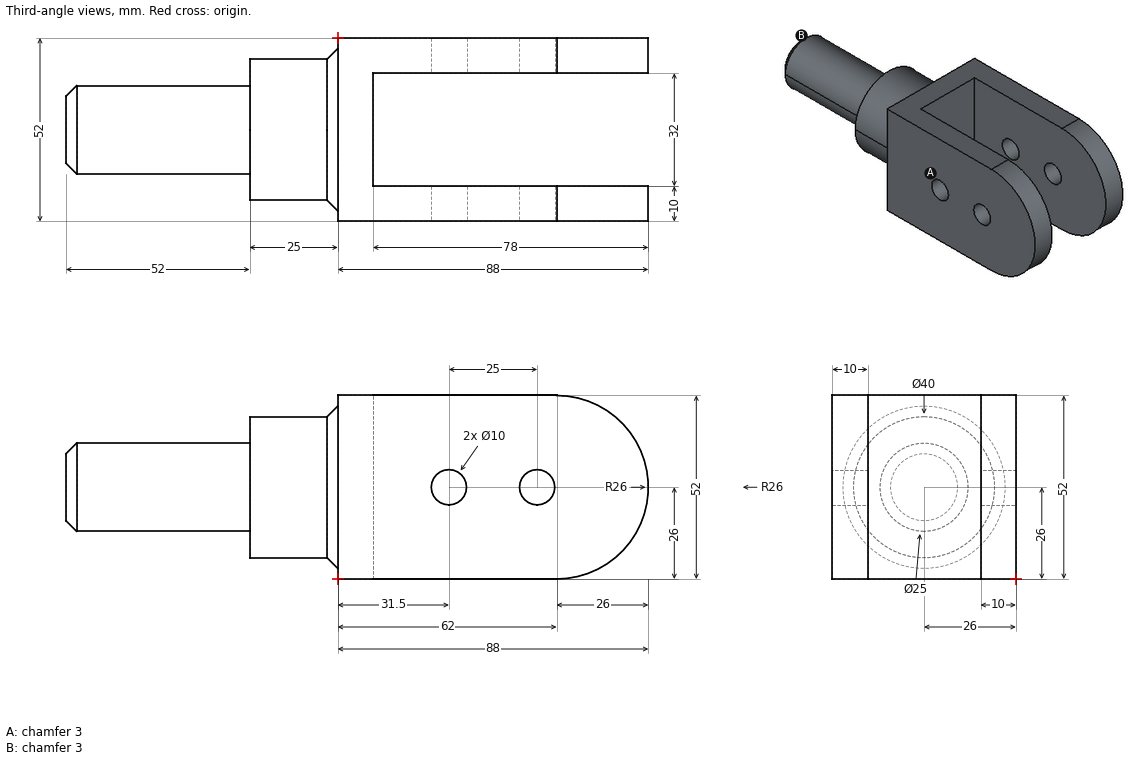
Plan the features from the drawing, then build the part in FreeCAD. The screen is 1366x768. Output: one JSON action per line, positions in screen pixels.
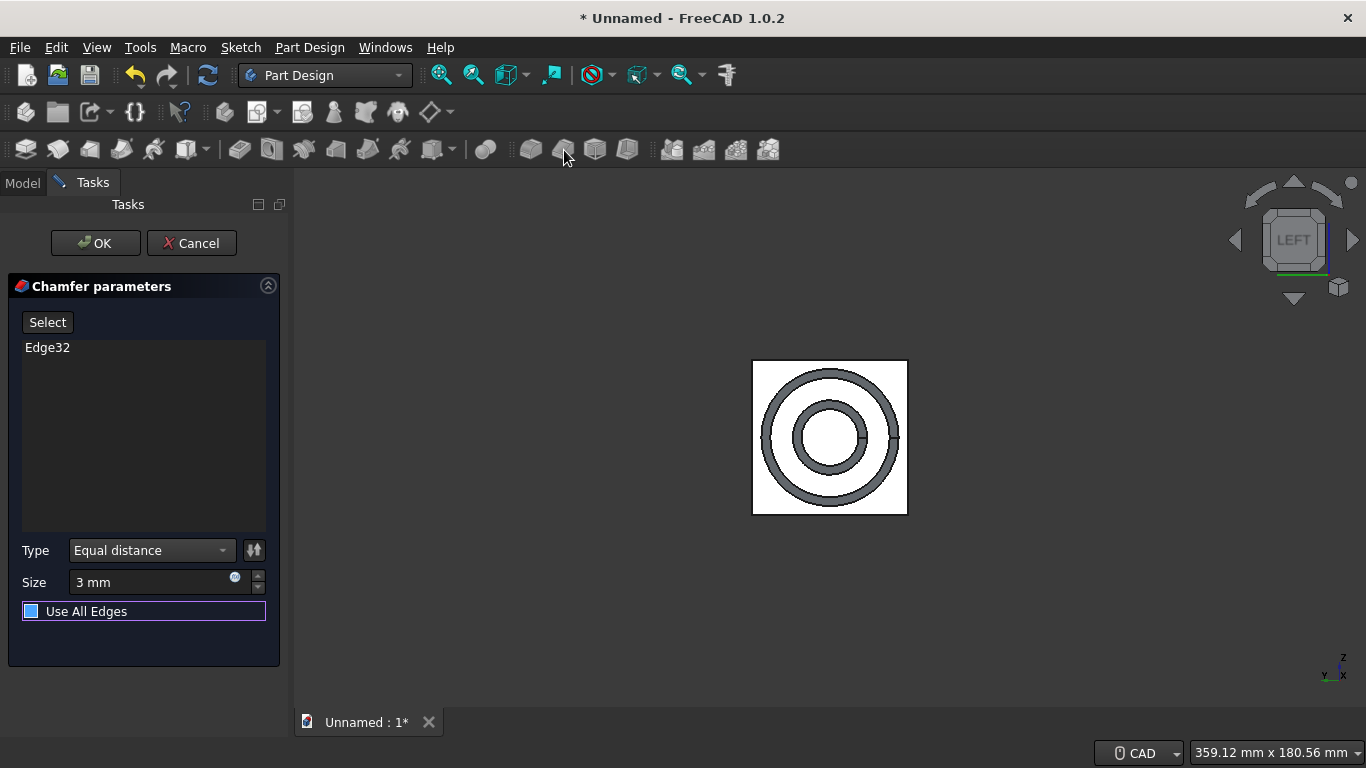
{"action": "left_click", "coordinate": [96, 243]}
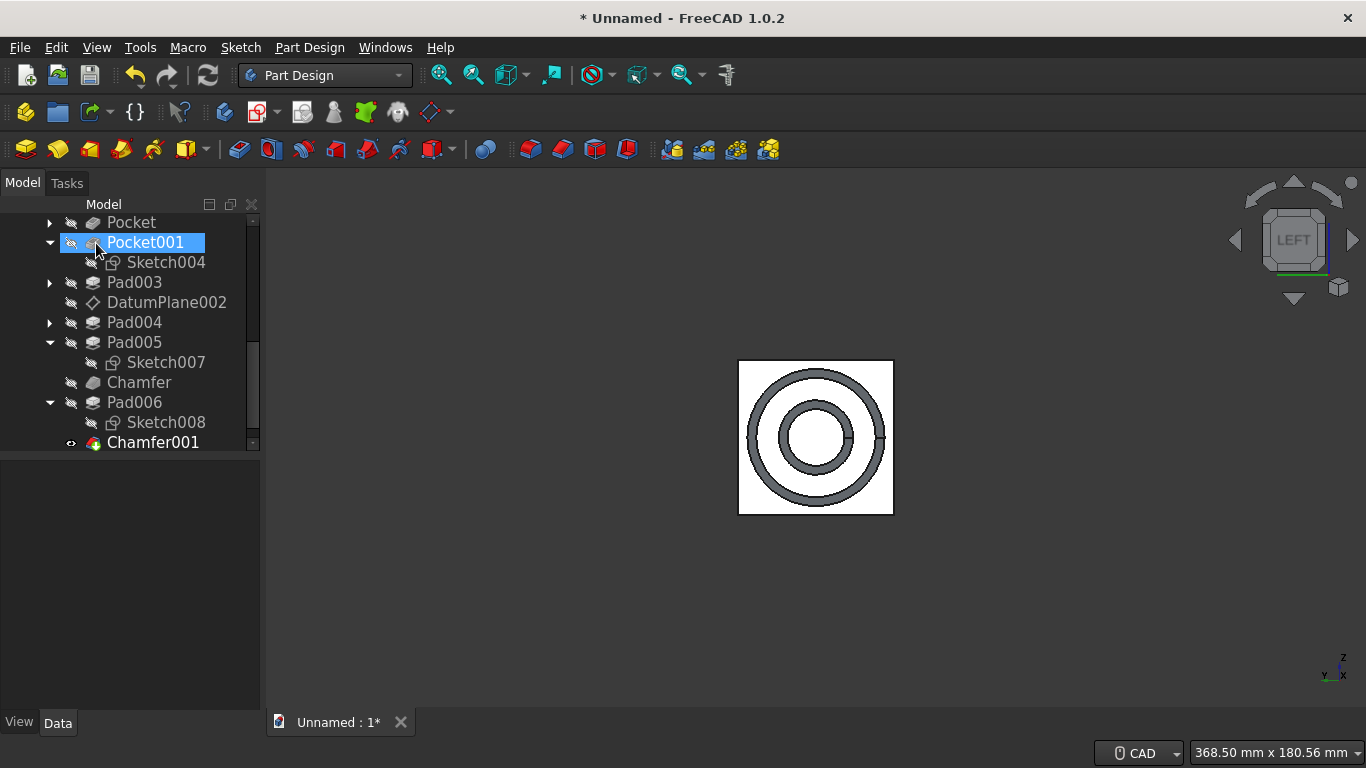
{"action": "left_click", "coordinate": [442, 76]}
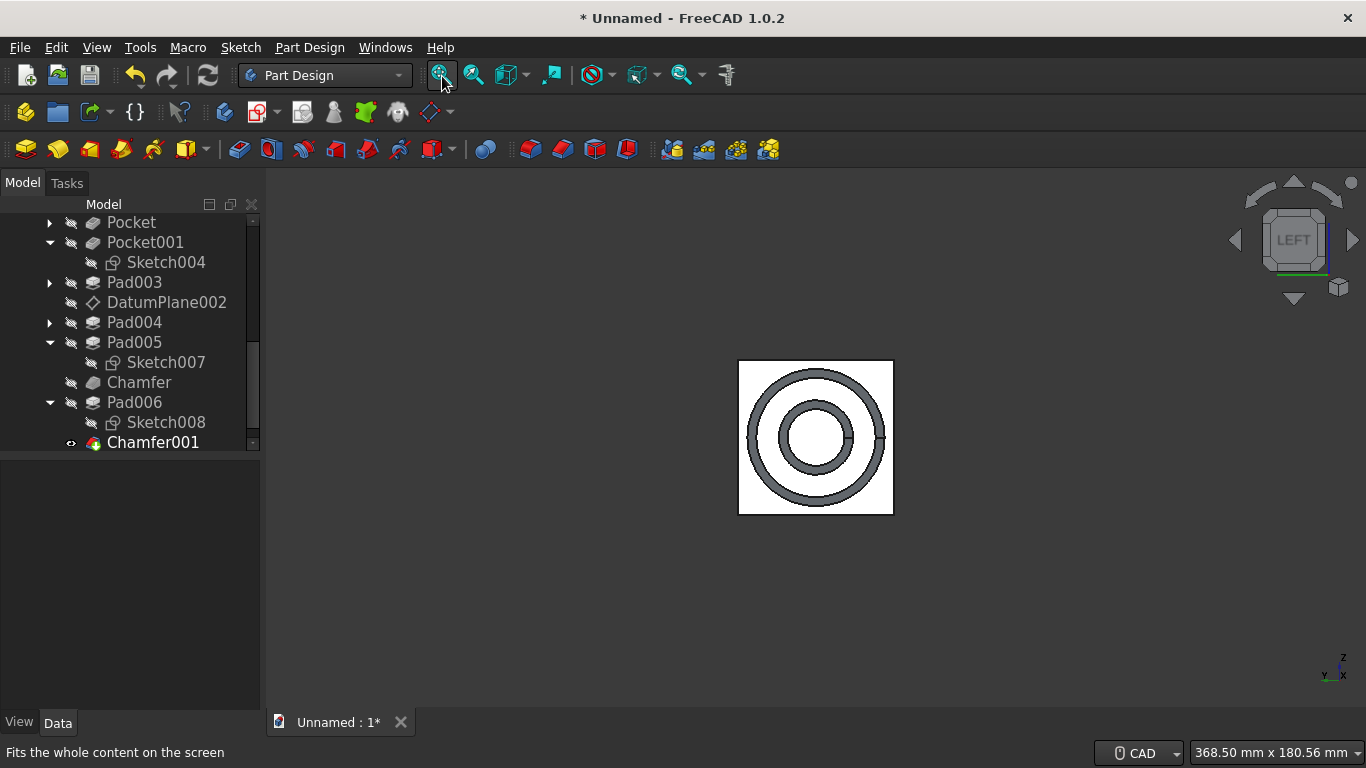
{"action": "key", "text": "0"}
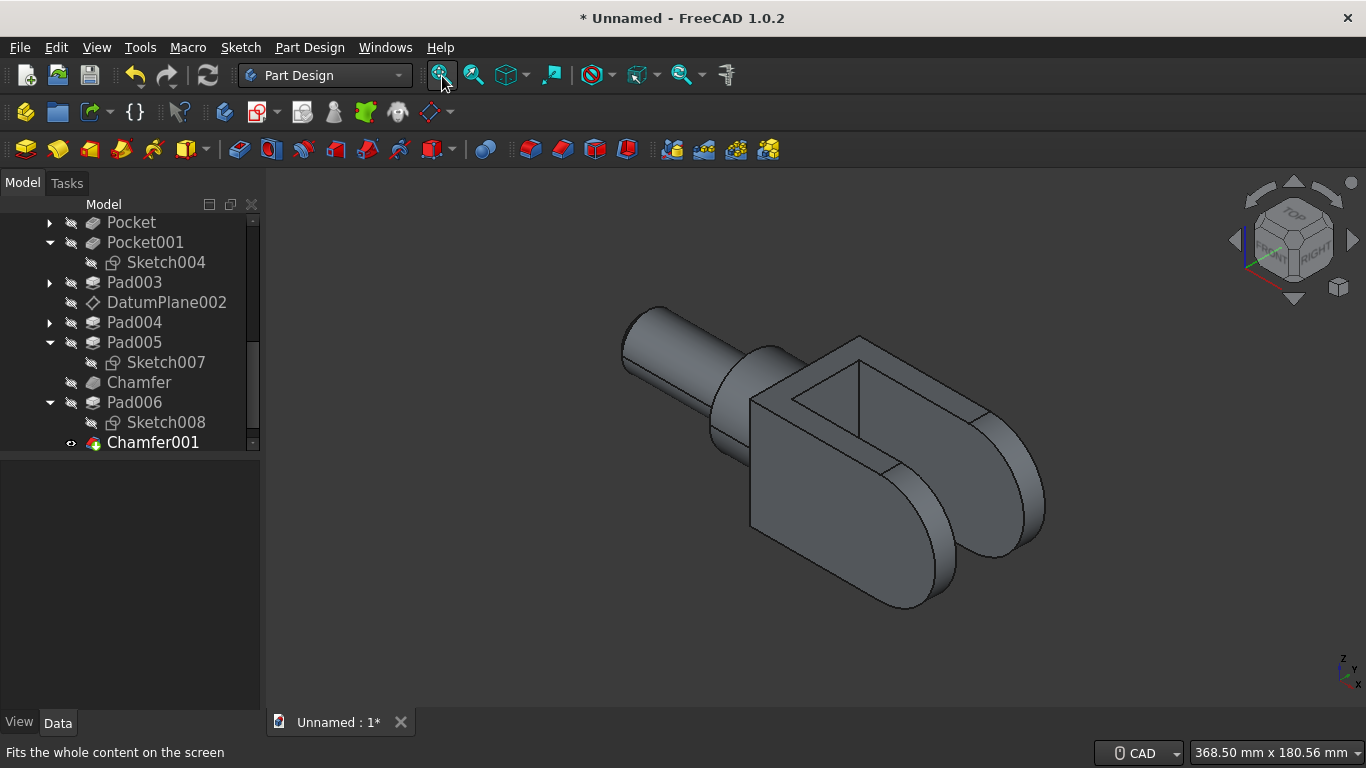
{"action": "left_click", "coordinate": [869, 530]}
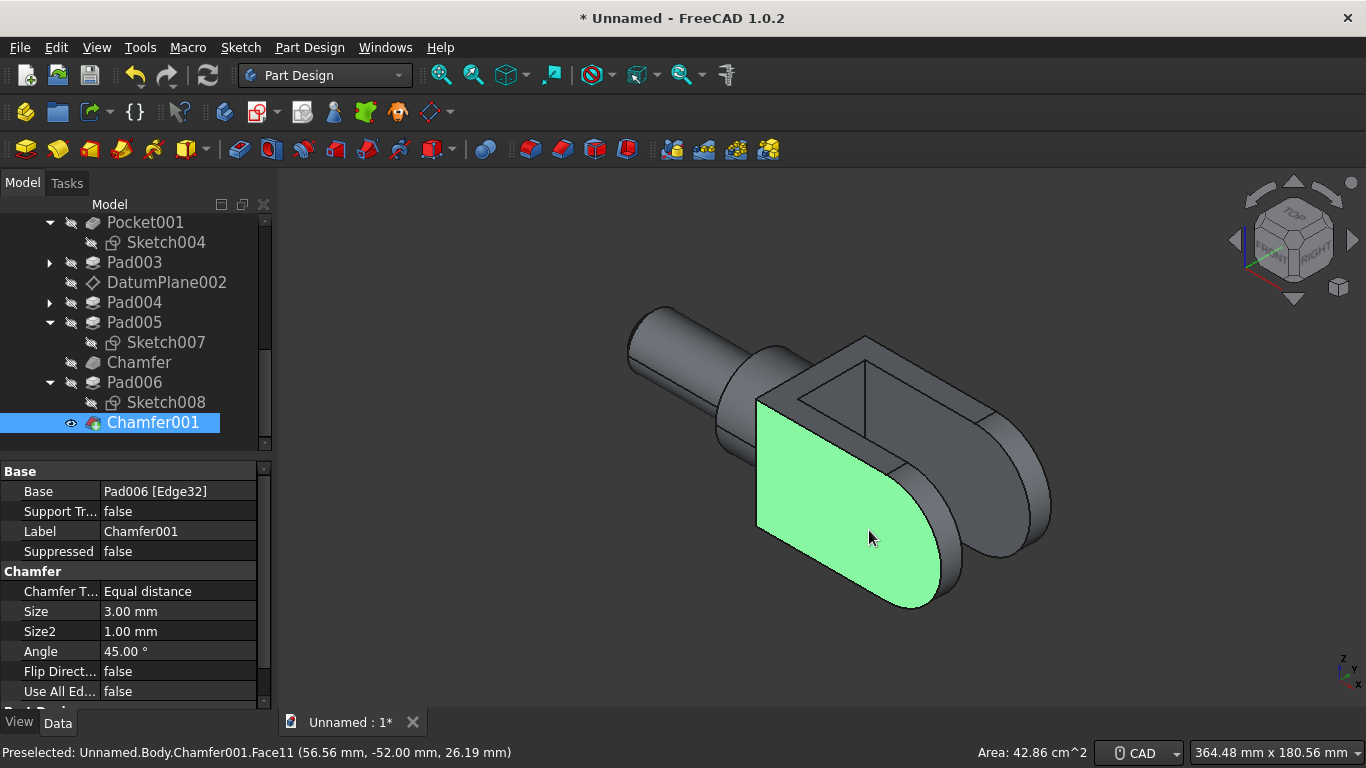
{"action": "left_click", "coordinate": [258, 112]}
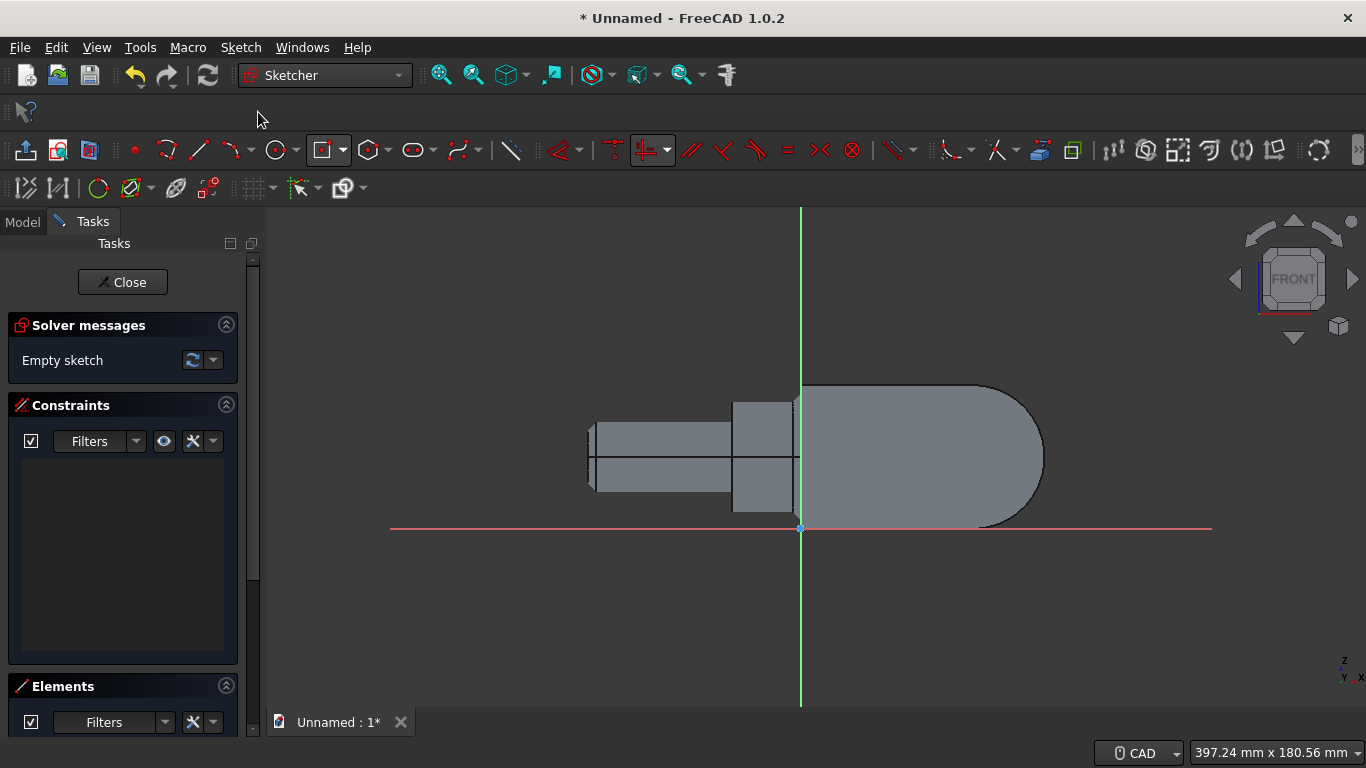
{"action": "scroll", "coordinate": [946, 499], "scroll_direction": "up", "scroll_amount": 6}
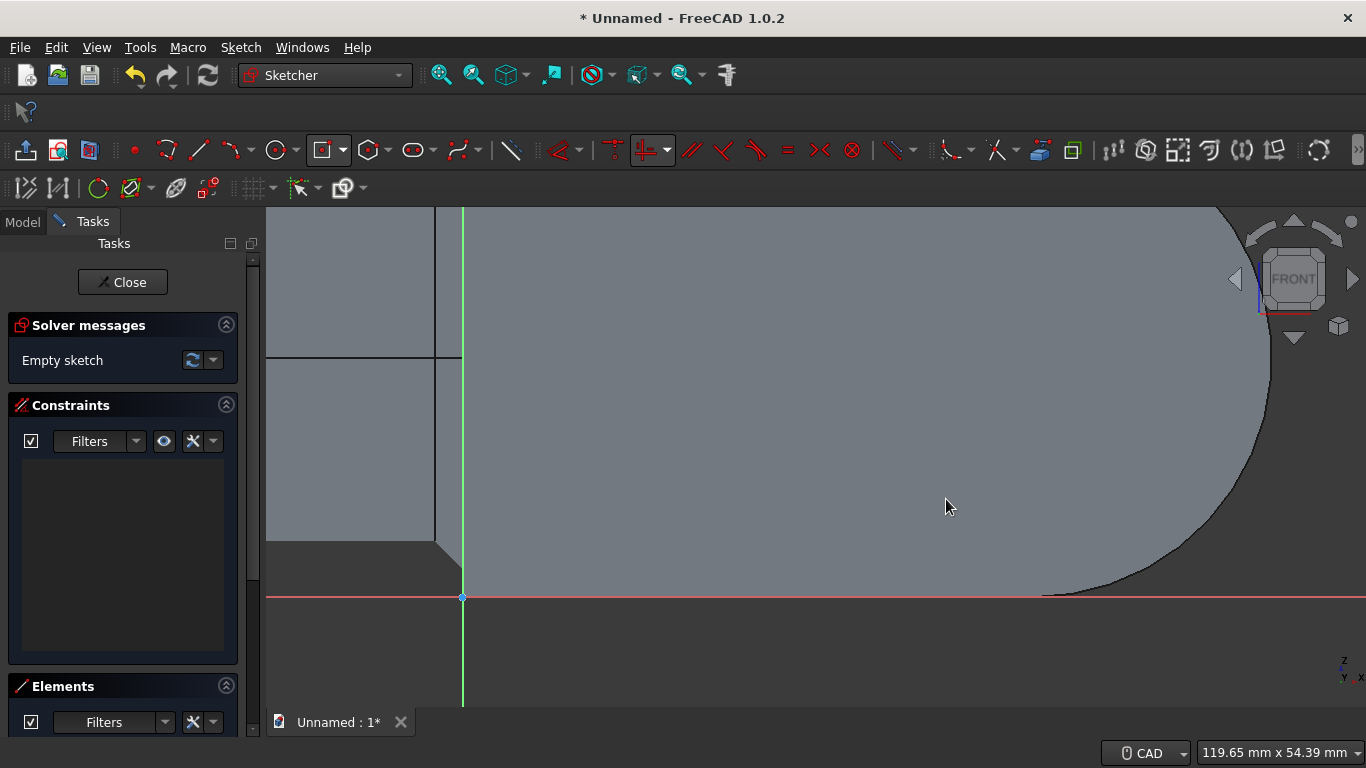
{"action": "left_click", "coordinate": [276, 150]}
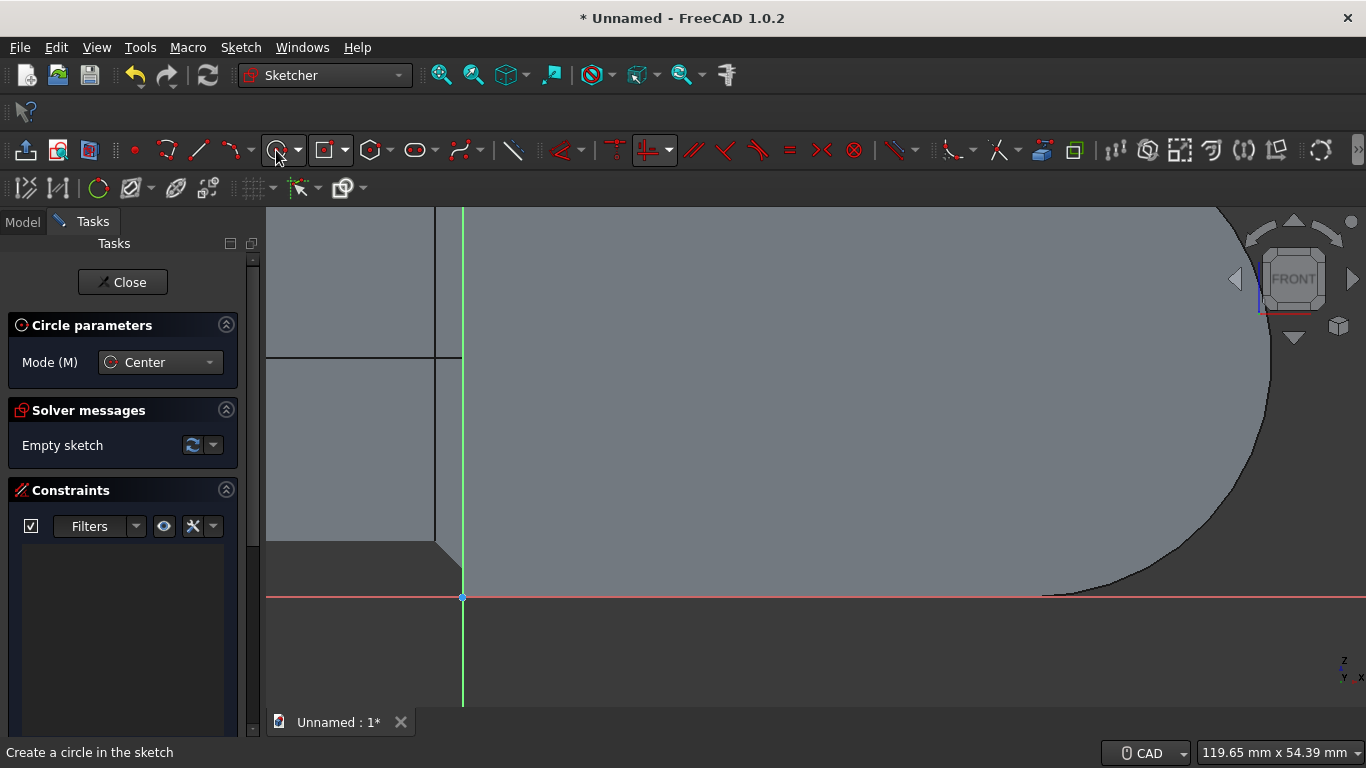
{"action": "left_click", "coordinate": [752, 358]}
{"action": "left_click", "coordinate": [785, 326]}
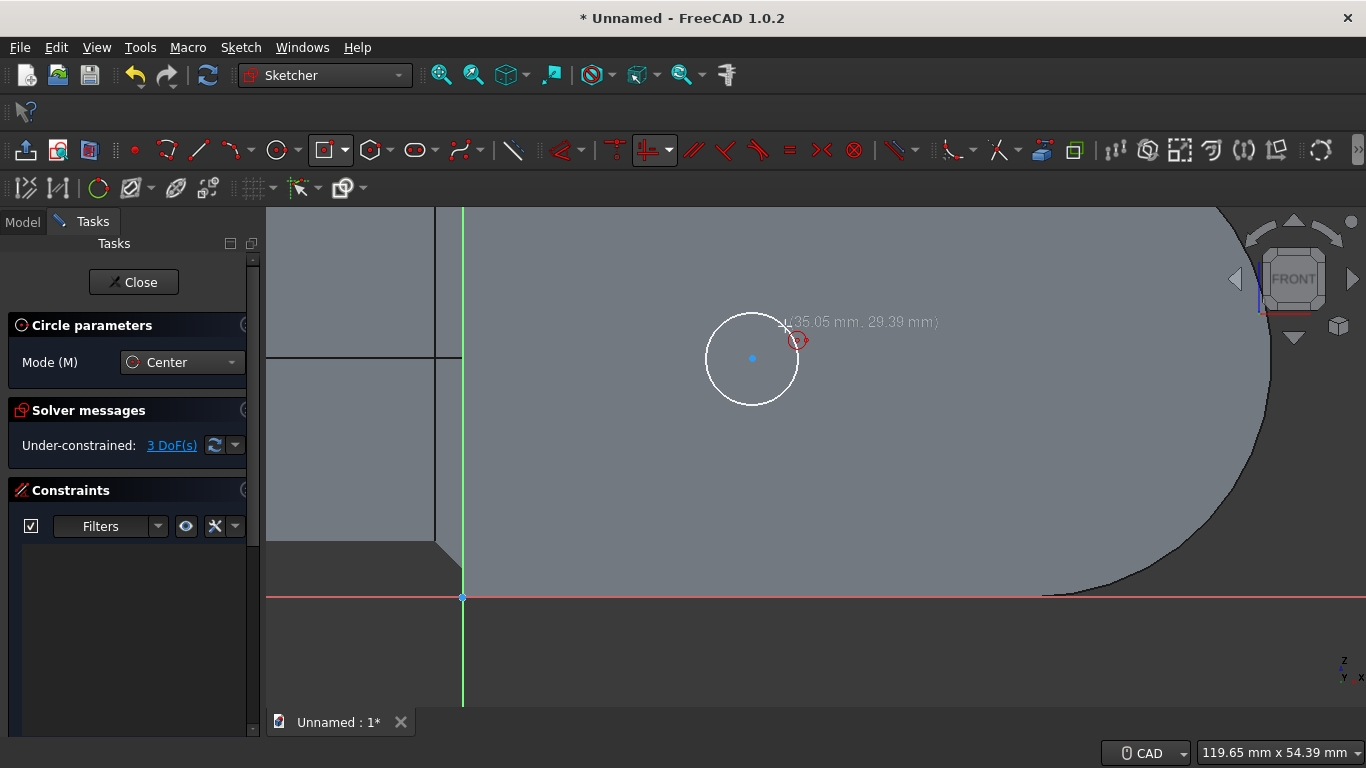
{"action": "left_click", "coordinate": [982, 358]}
{"action": "left_click", "coordinate": [1015, 326]}
{"action": "key", "text": "Escape"}